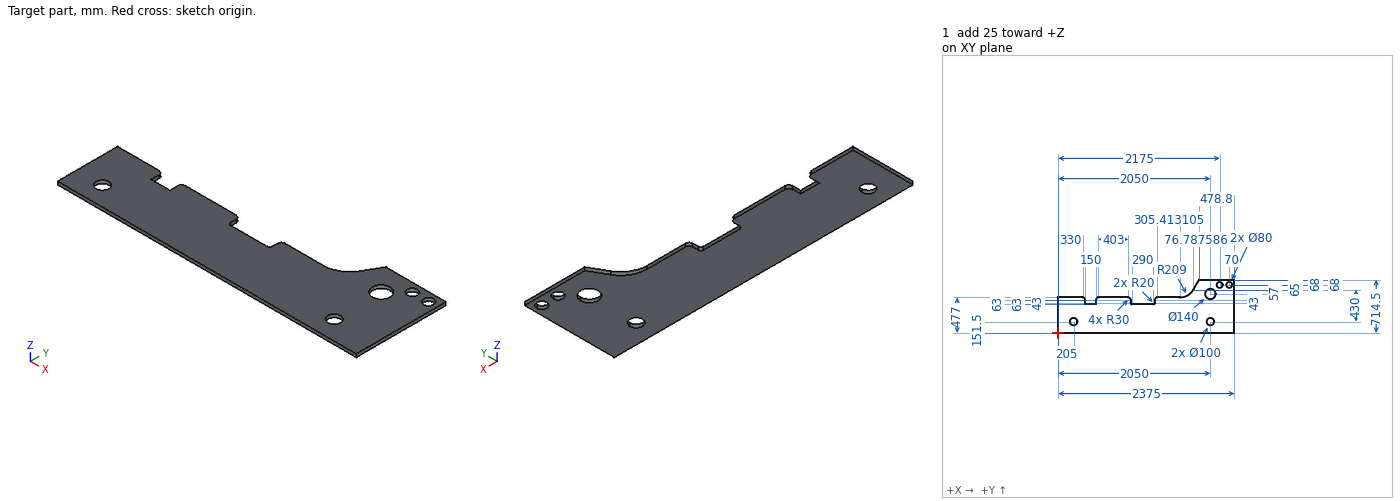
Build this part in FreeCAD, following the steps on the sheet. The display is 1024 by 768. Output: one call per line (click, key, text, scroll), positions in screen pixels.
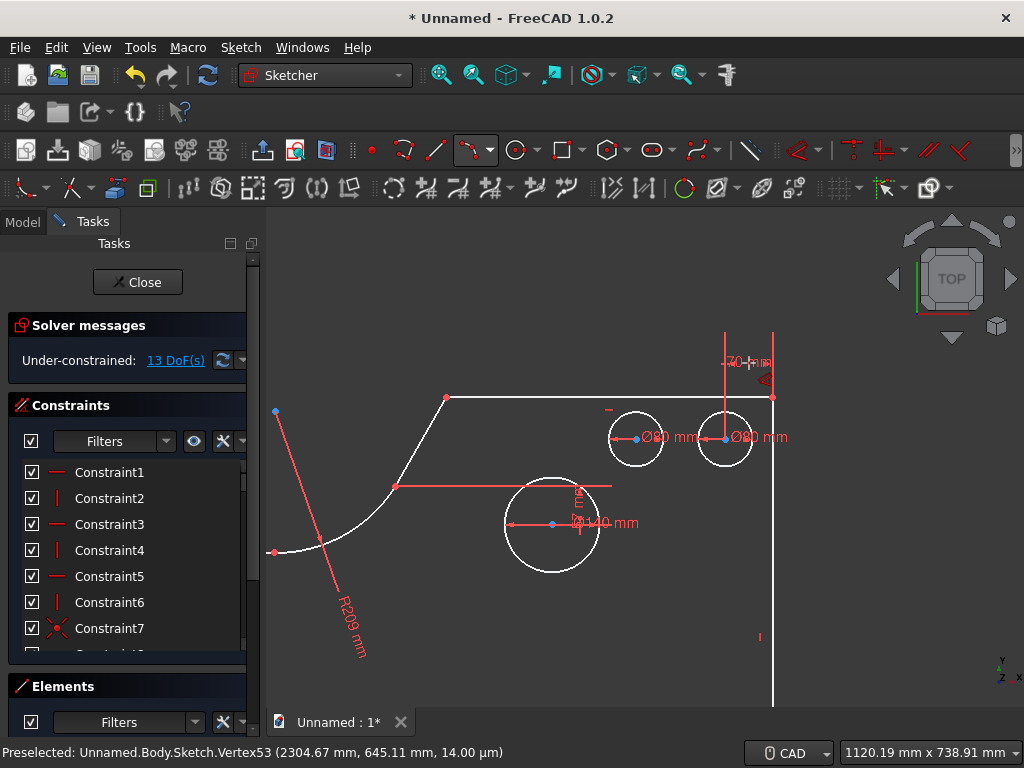
click(773, 397)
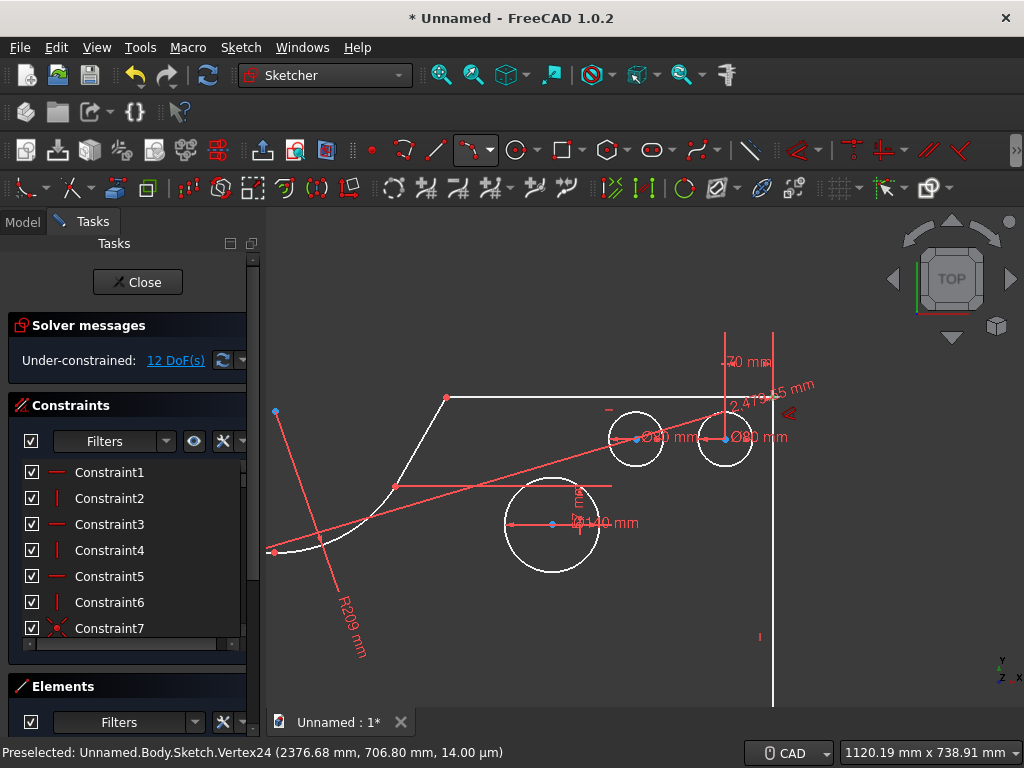
click(725, 439)
click(807, 418)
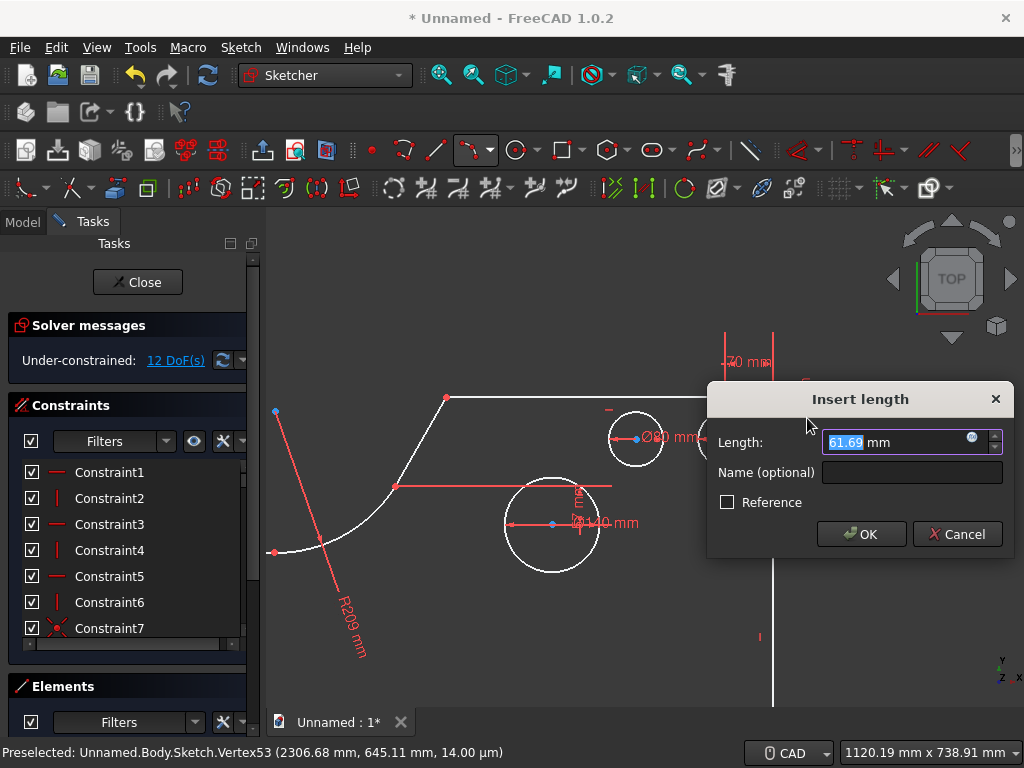
text(68)
key(Return)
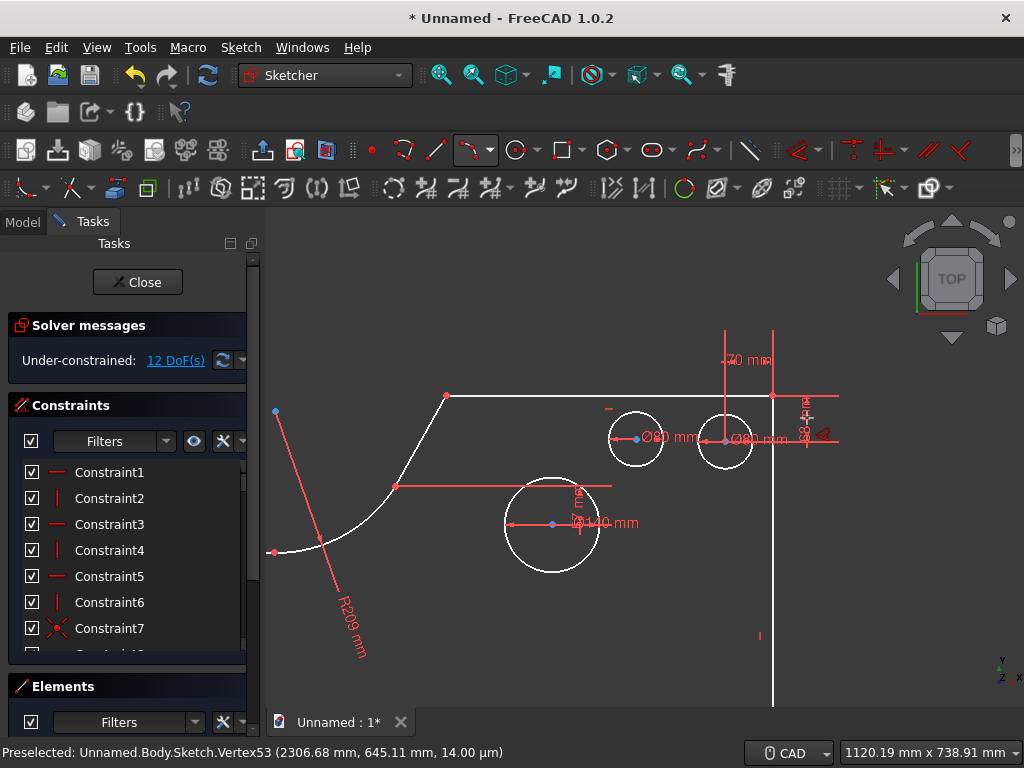
click(395, 486)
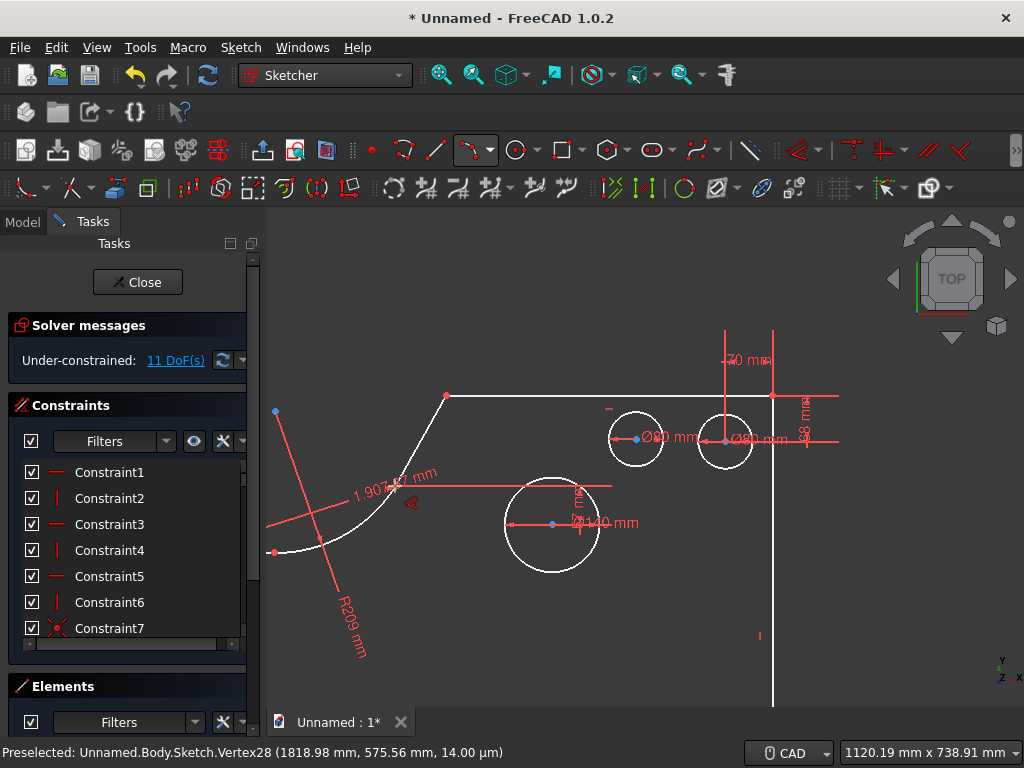
click(725, 442)
click(759, 464)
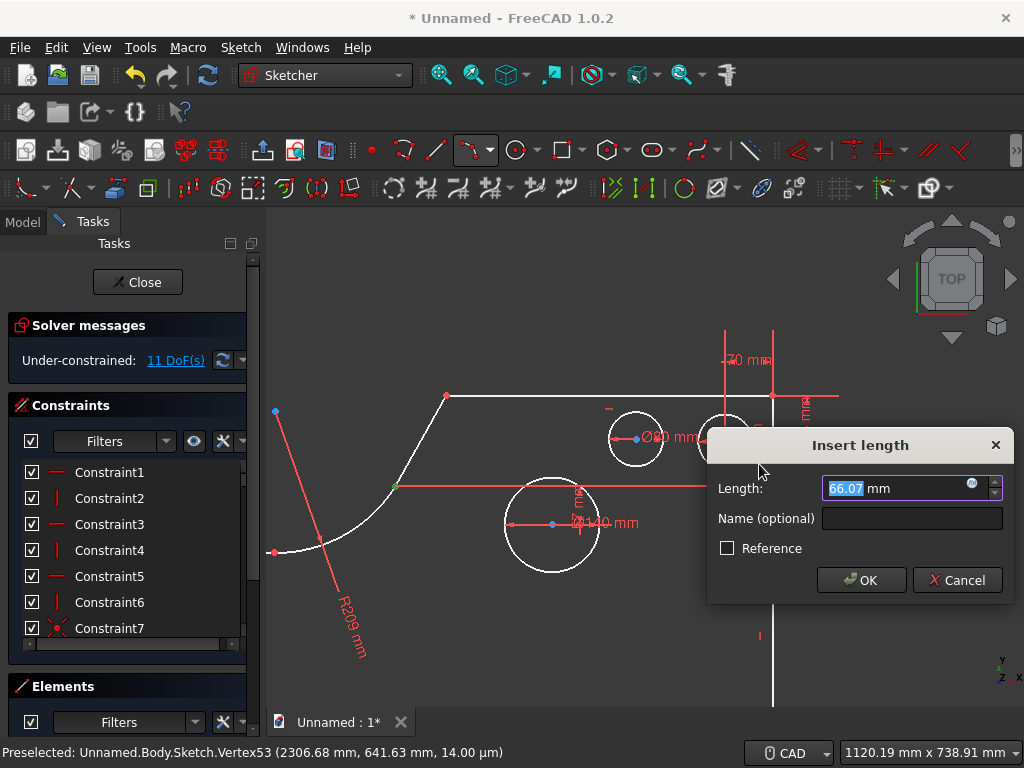
text(65)
key(Return)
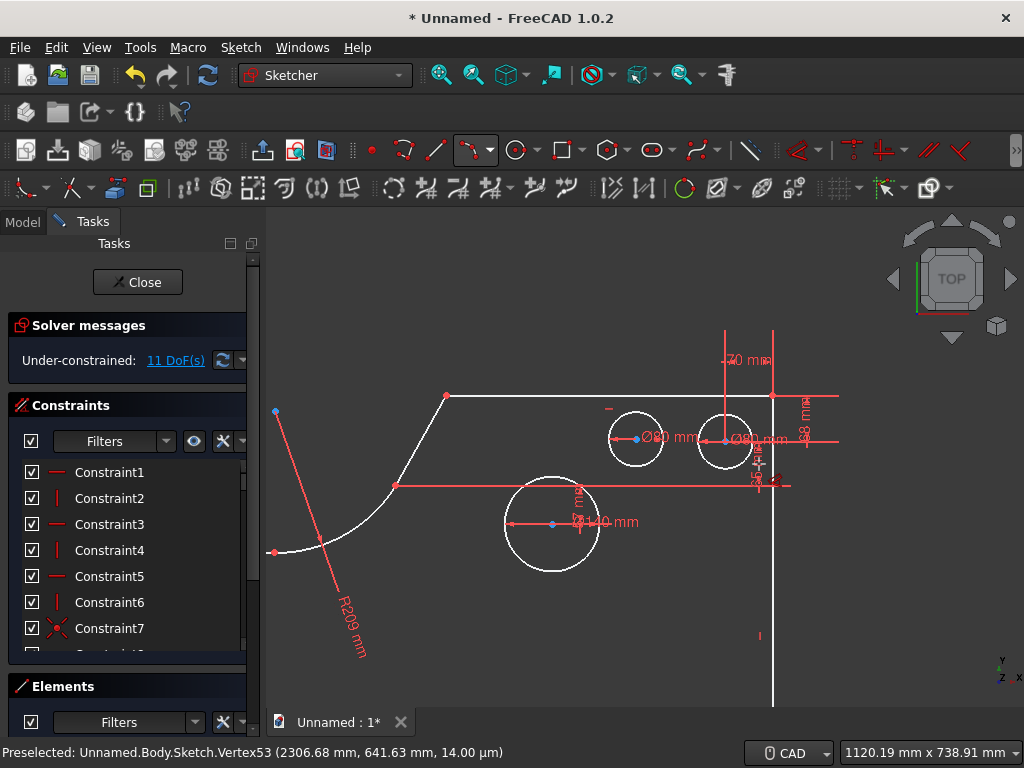
click(773, 396)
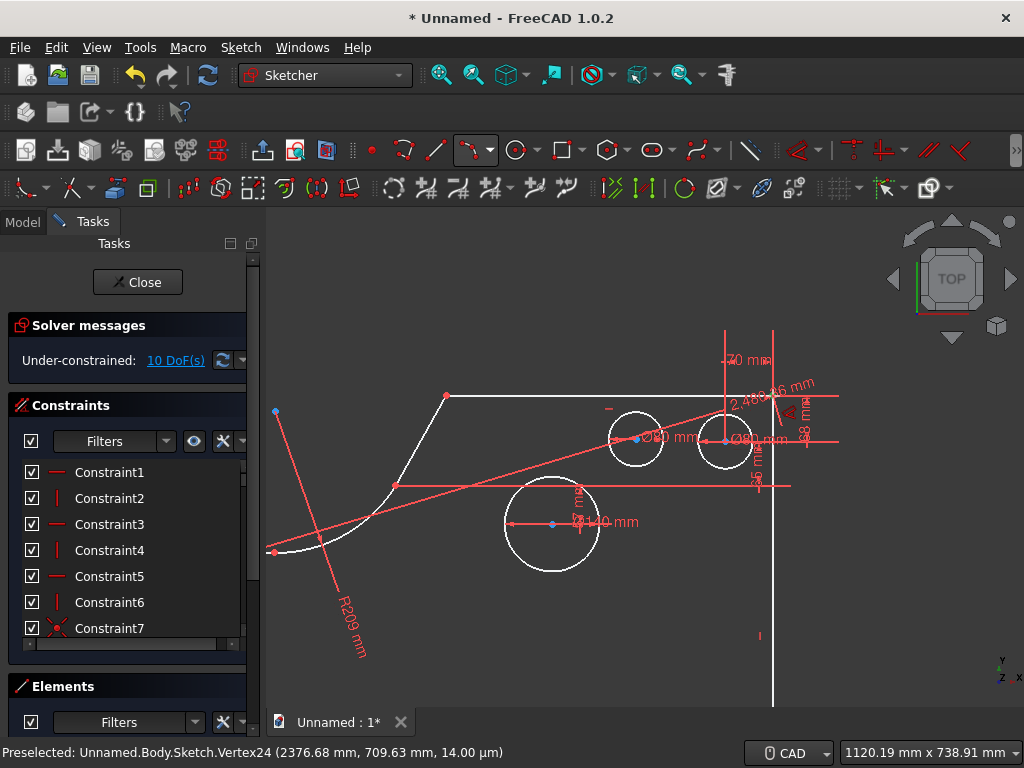
click(636, 439)
click(602, 417)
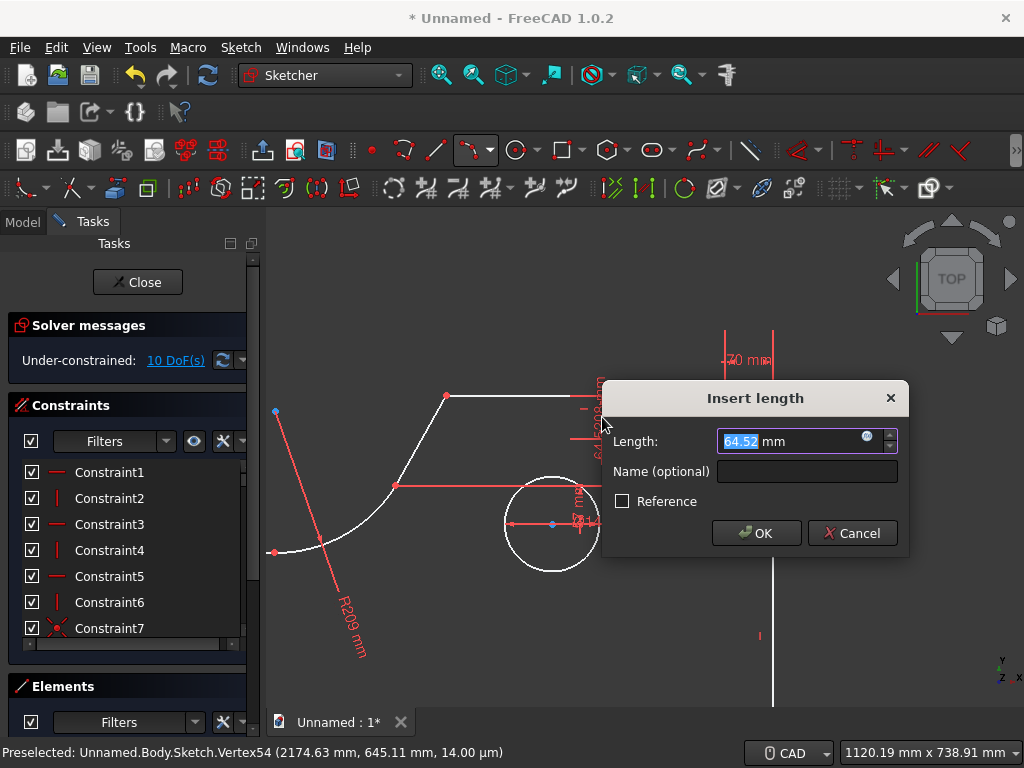
text(68)
key(Return)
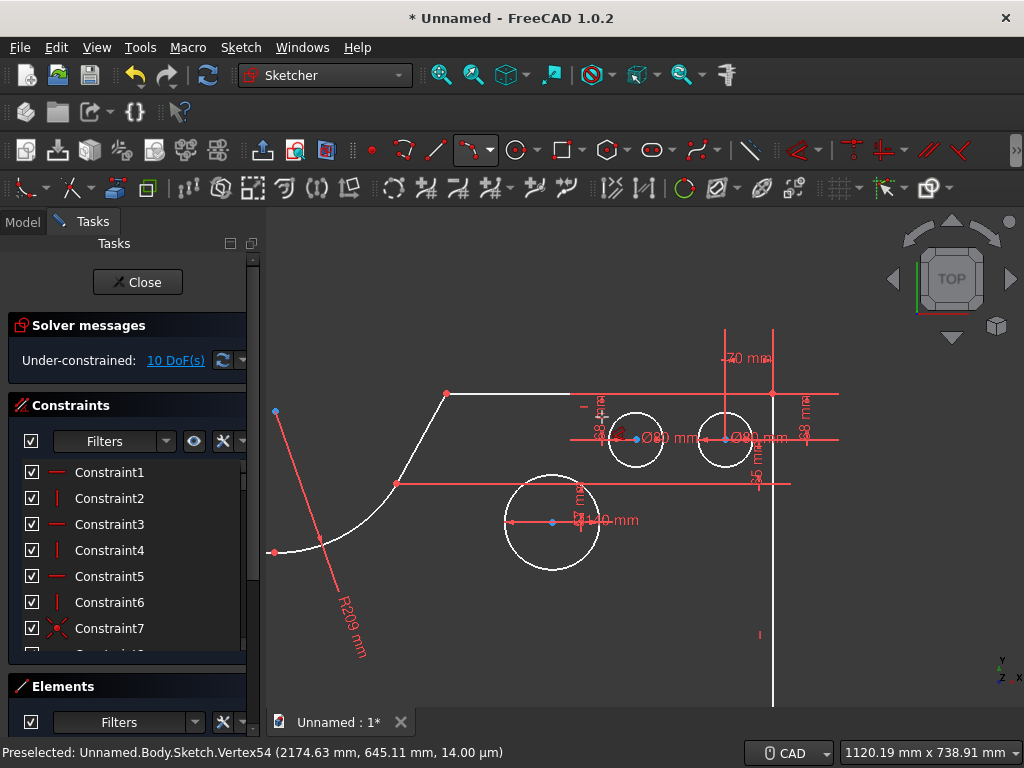
scroll(776, 399, down, 7)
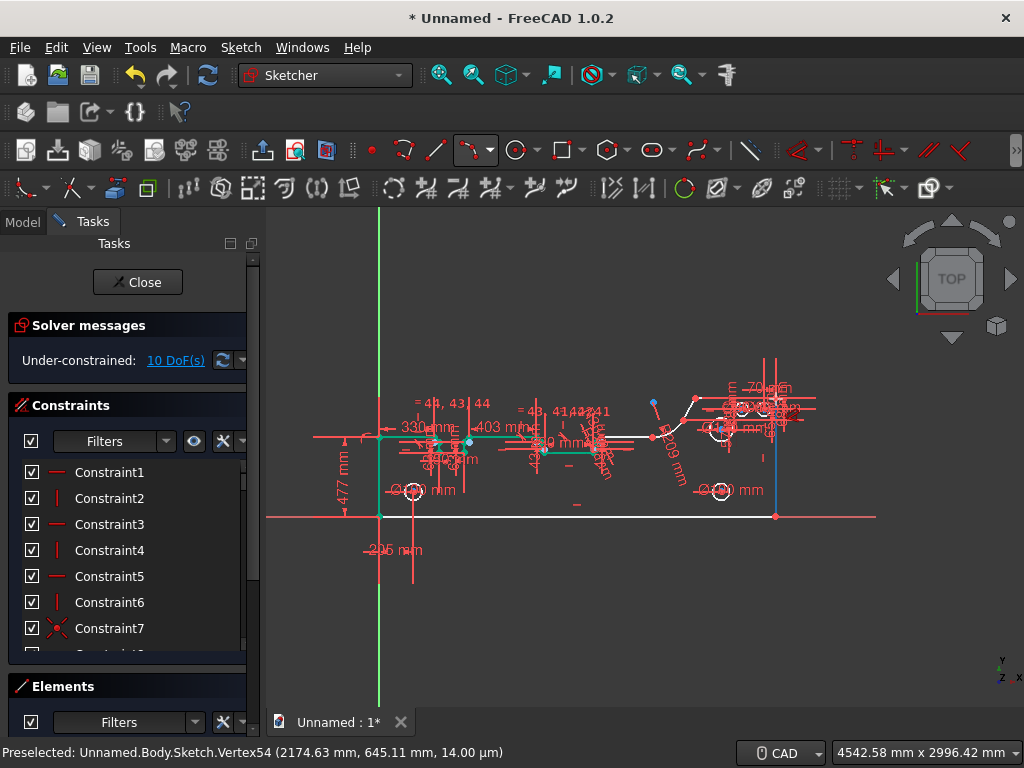
click(498, 517)
click(577, 551)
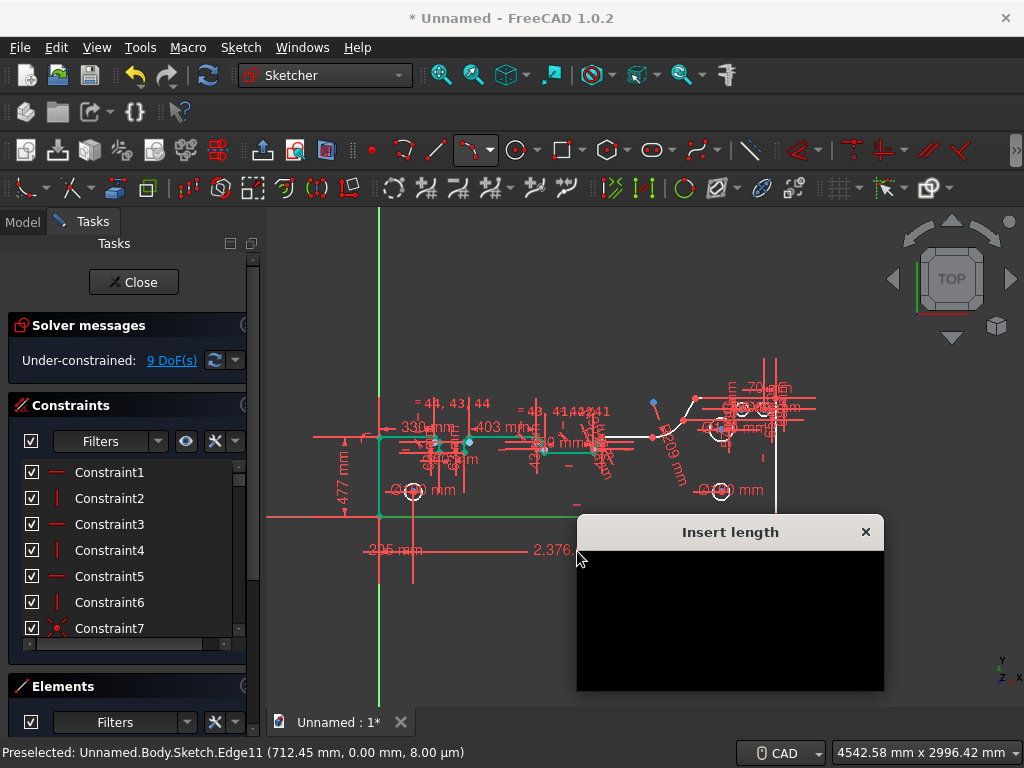
text(2375)
key(Return)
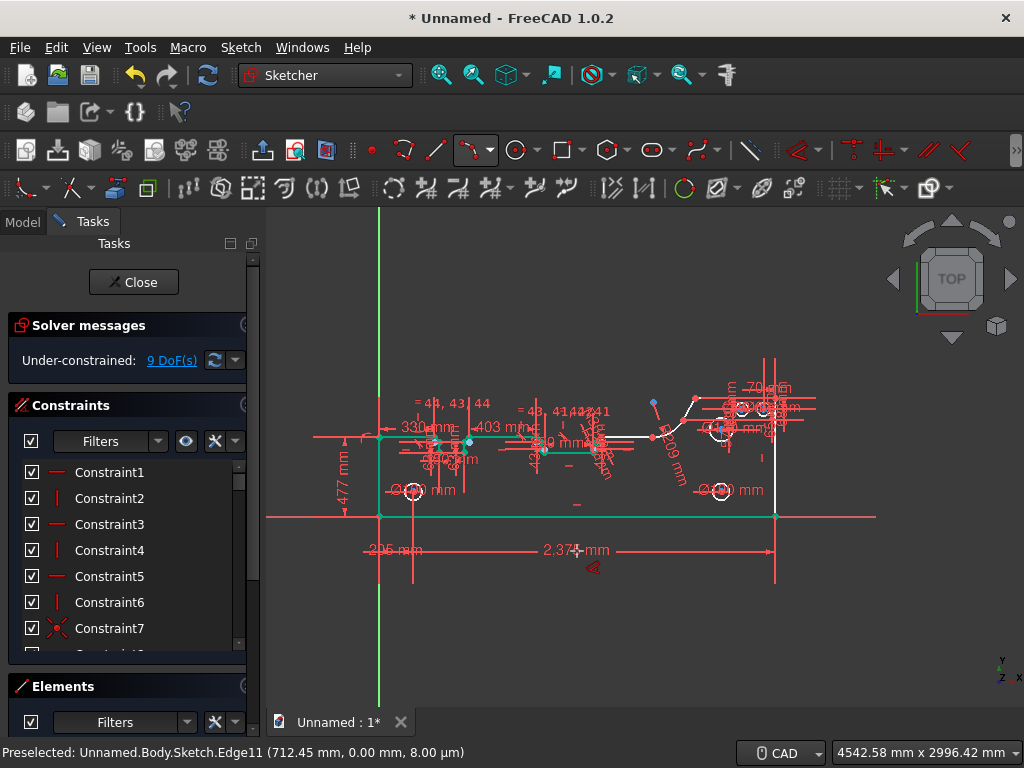
click(721, 492)
click(471, 551)